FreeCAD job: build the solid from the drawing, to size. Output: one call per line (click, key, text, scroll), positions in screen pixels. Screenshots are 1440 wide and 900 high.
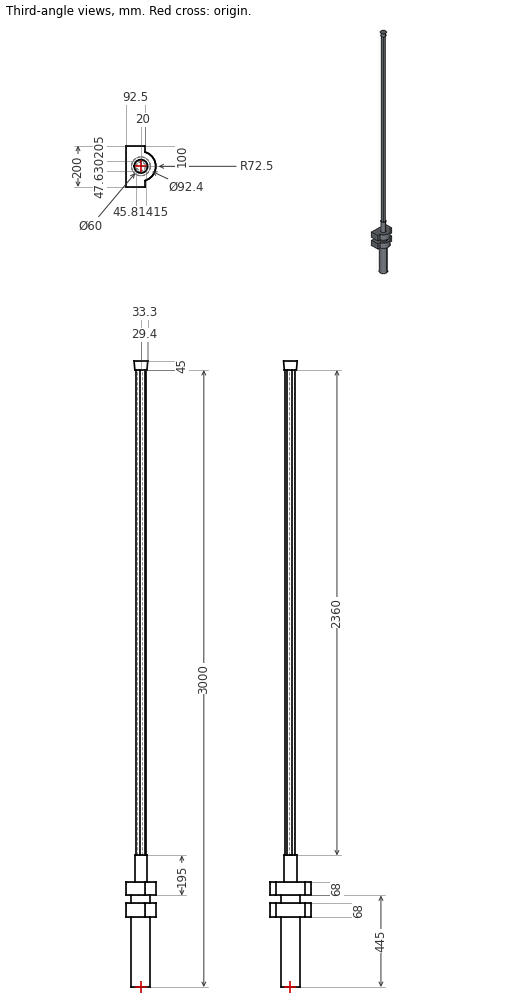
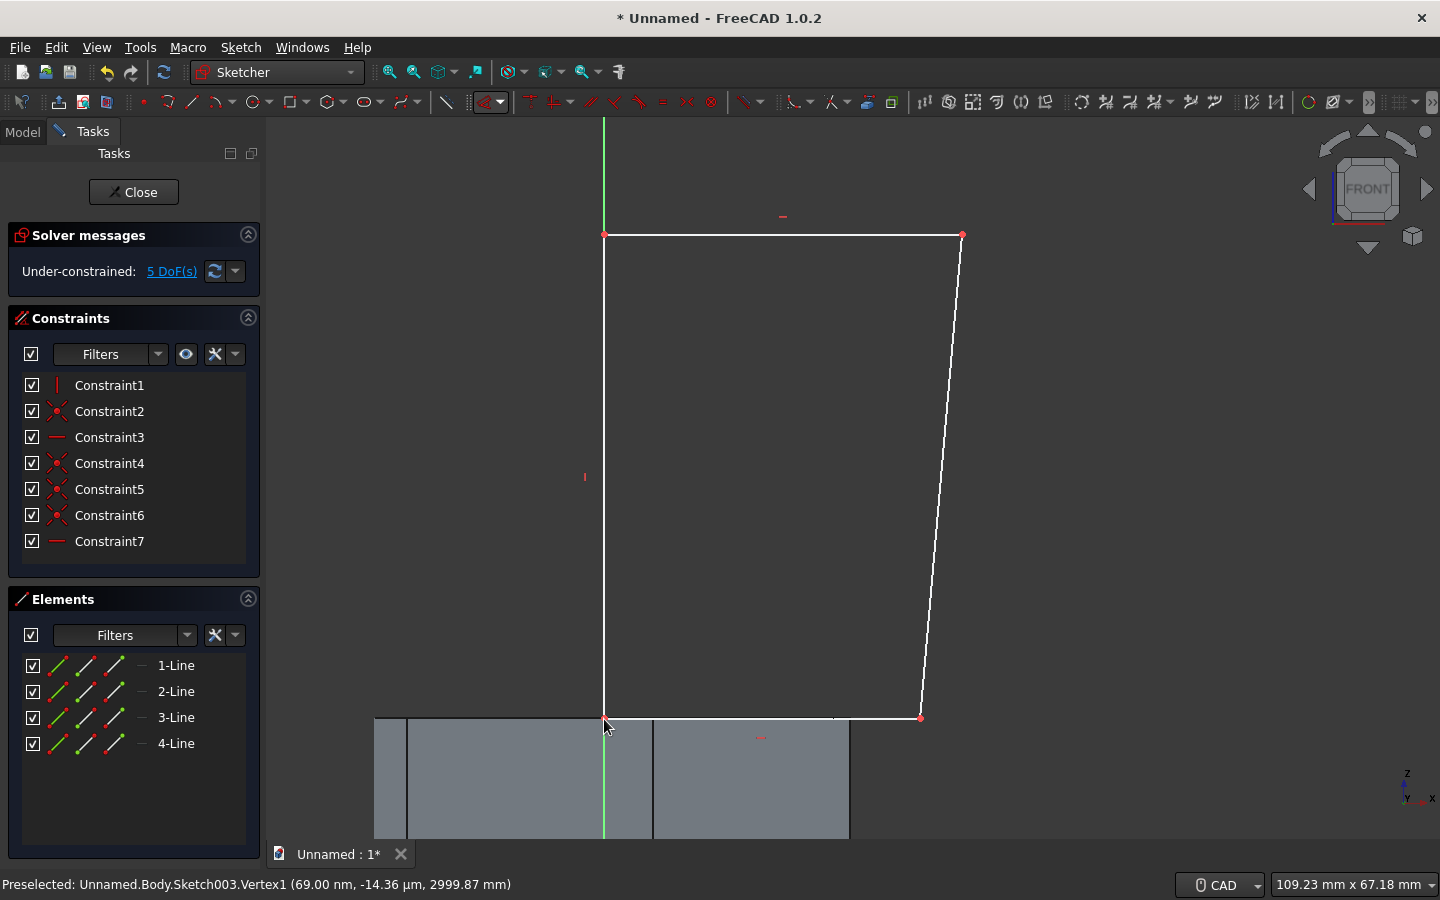
click(604, 719)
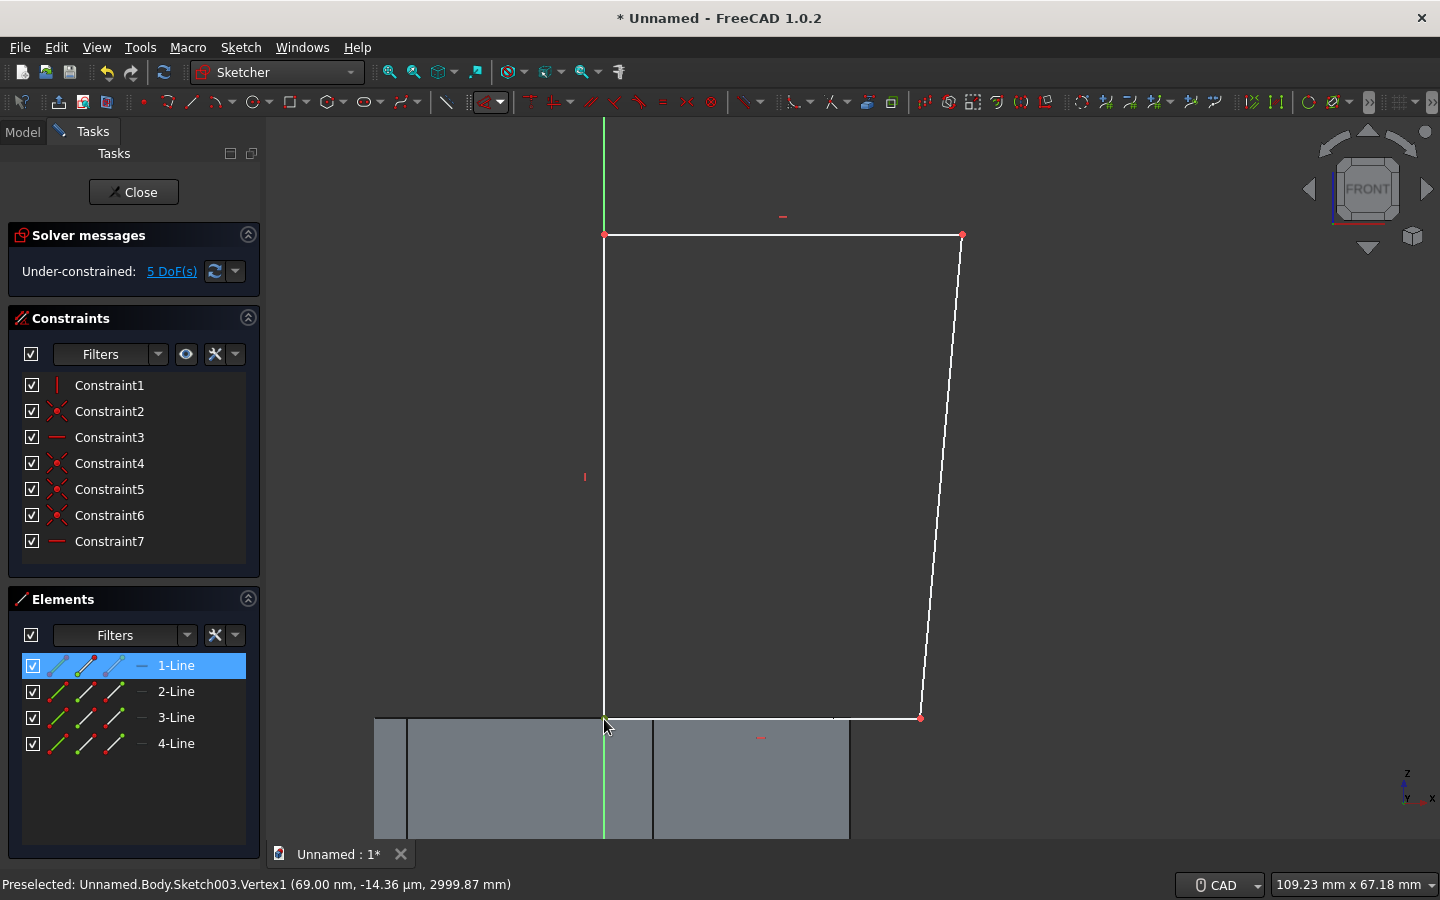
click(604, 763)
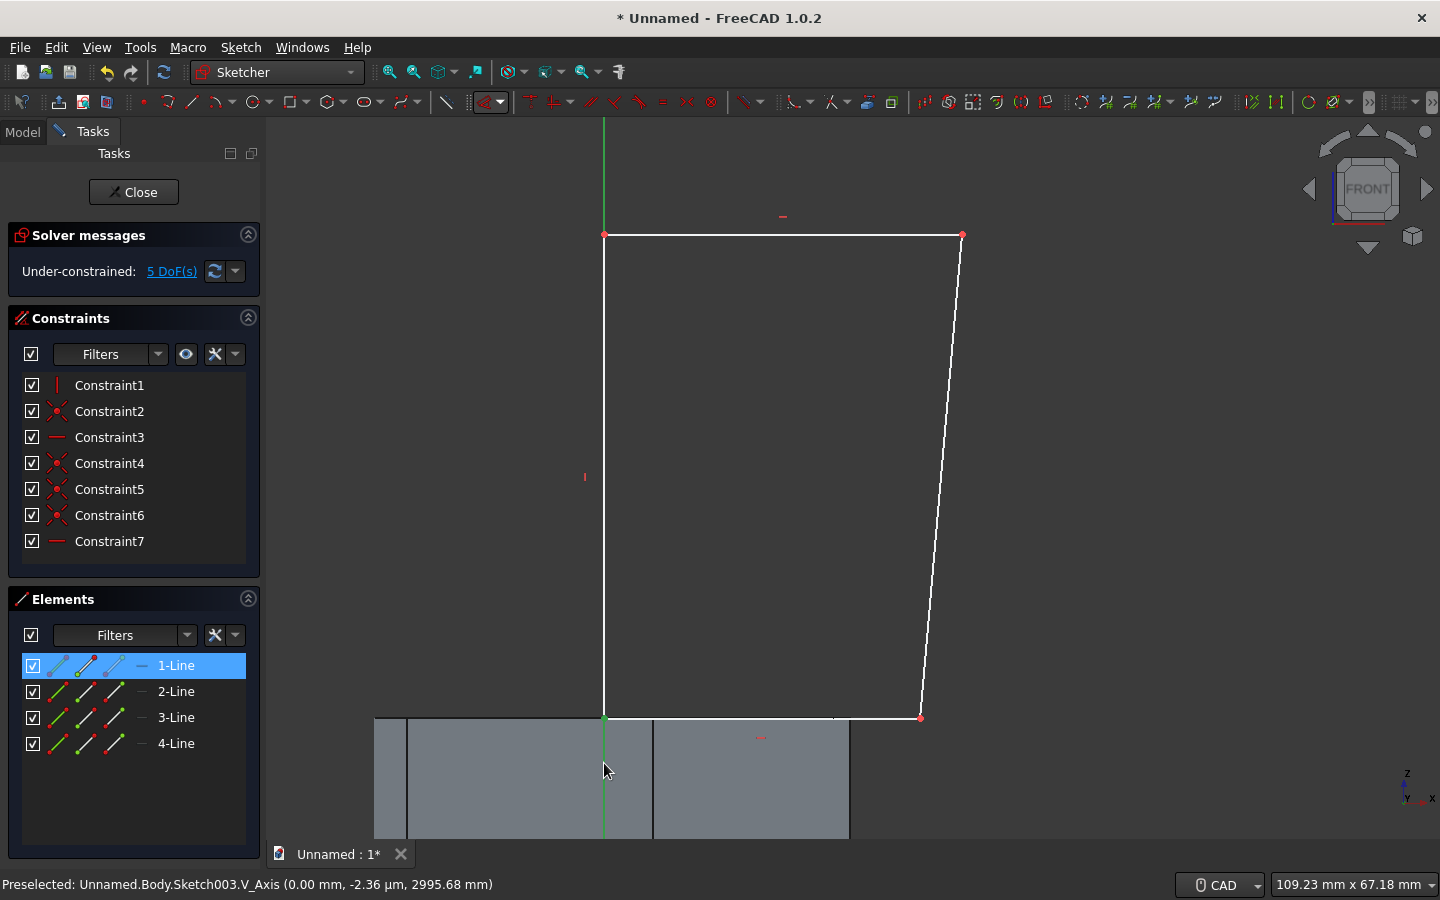
key(c)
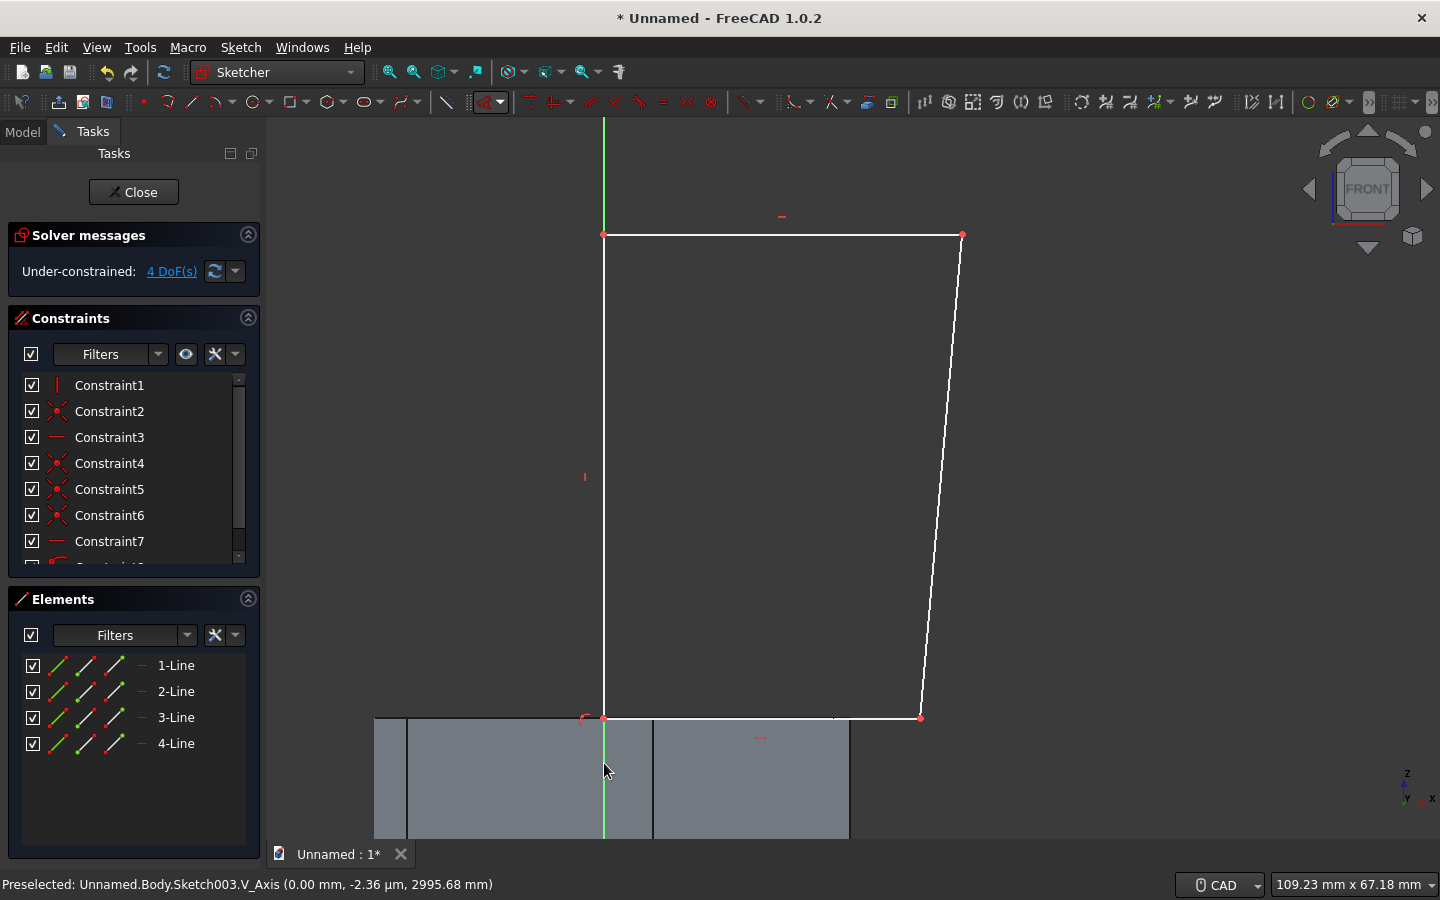
click(604, 574)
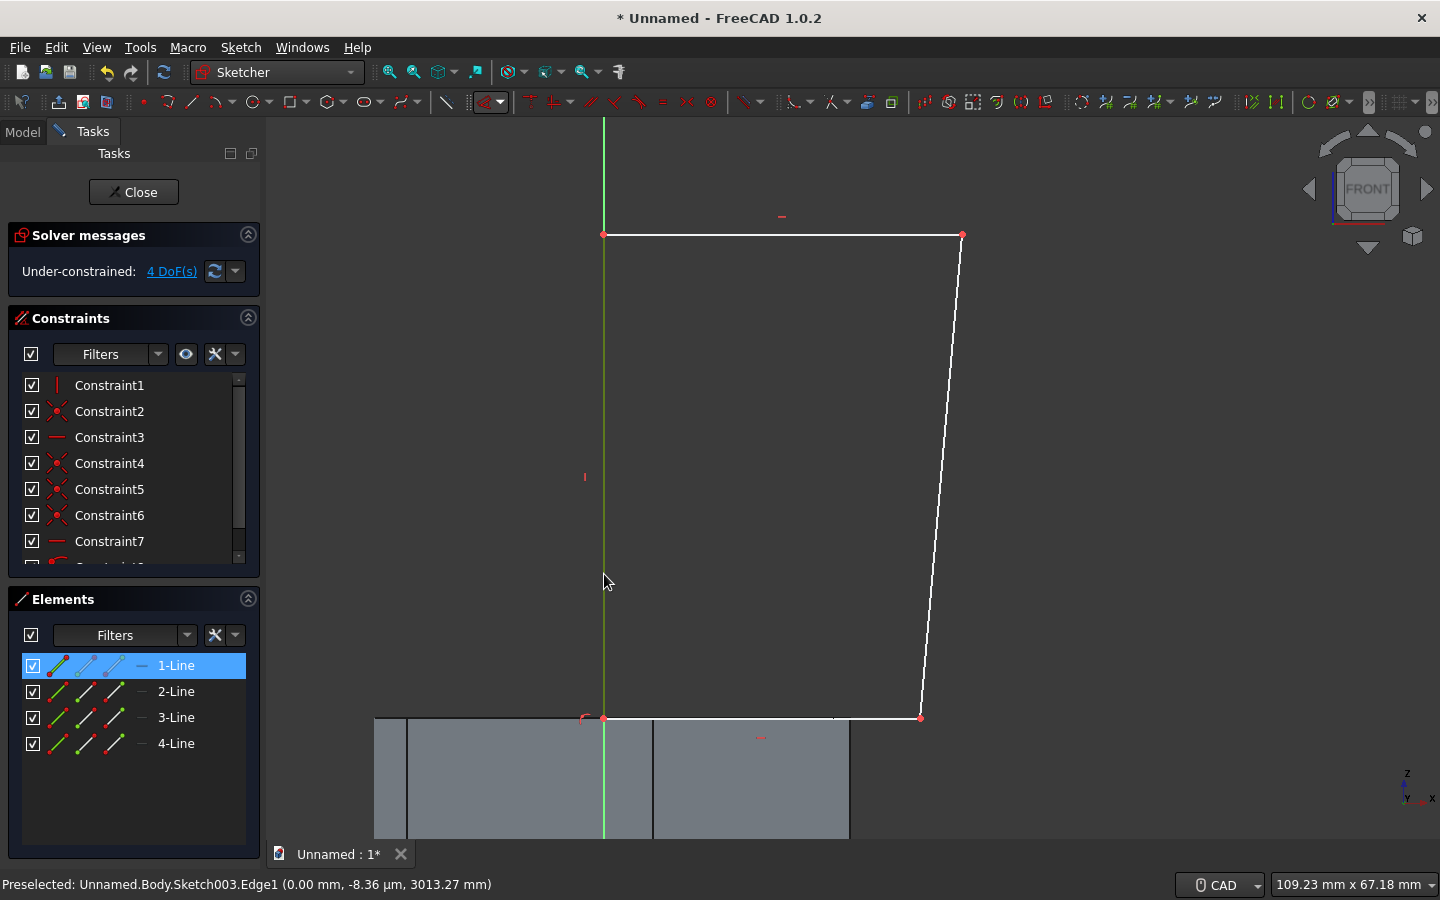
key(i)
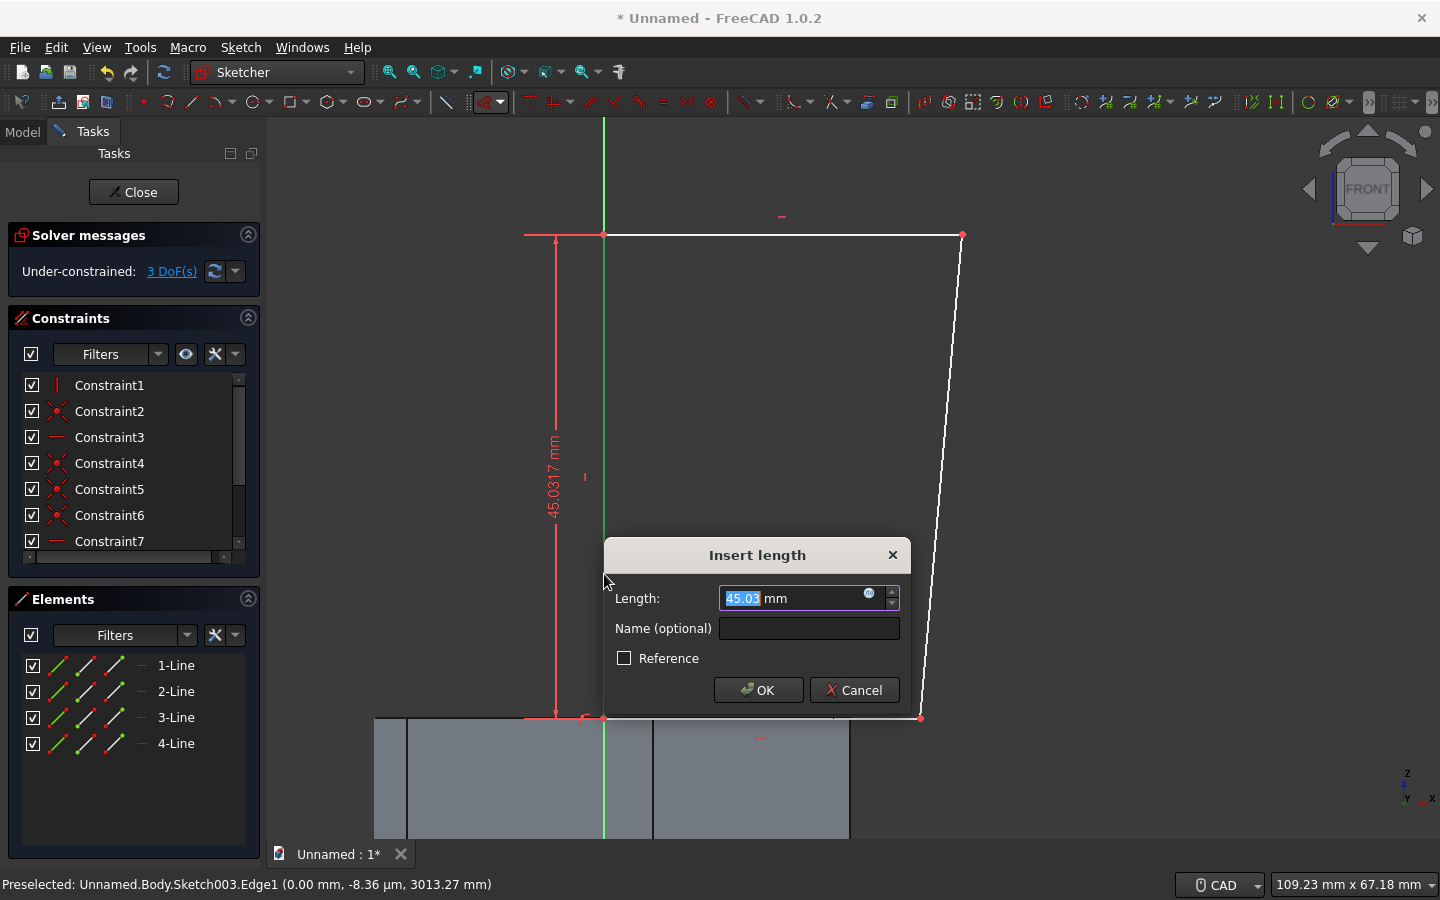
text(45)
key(Return)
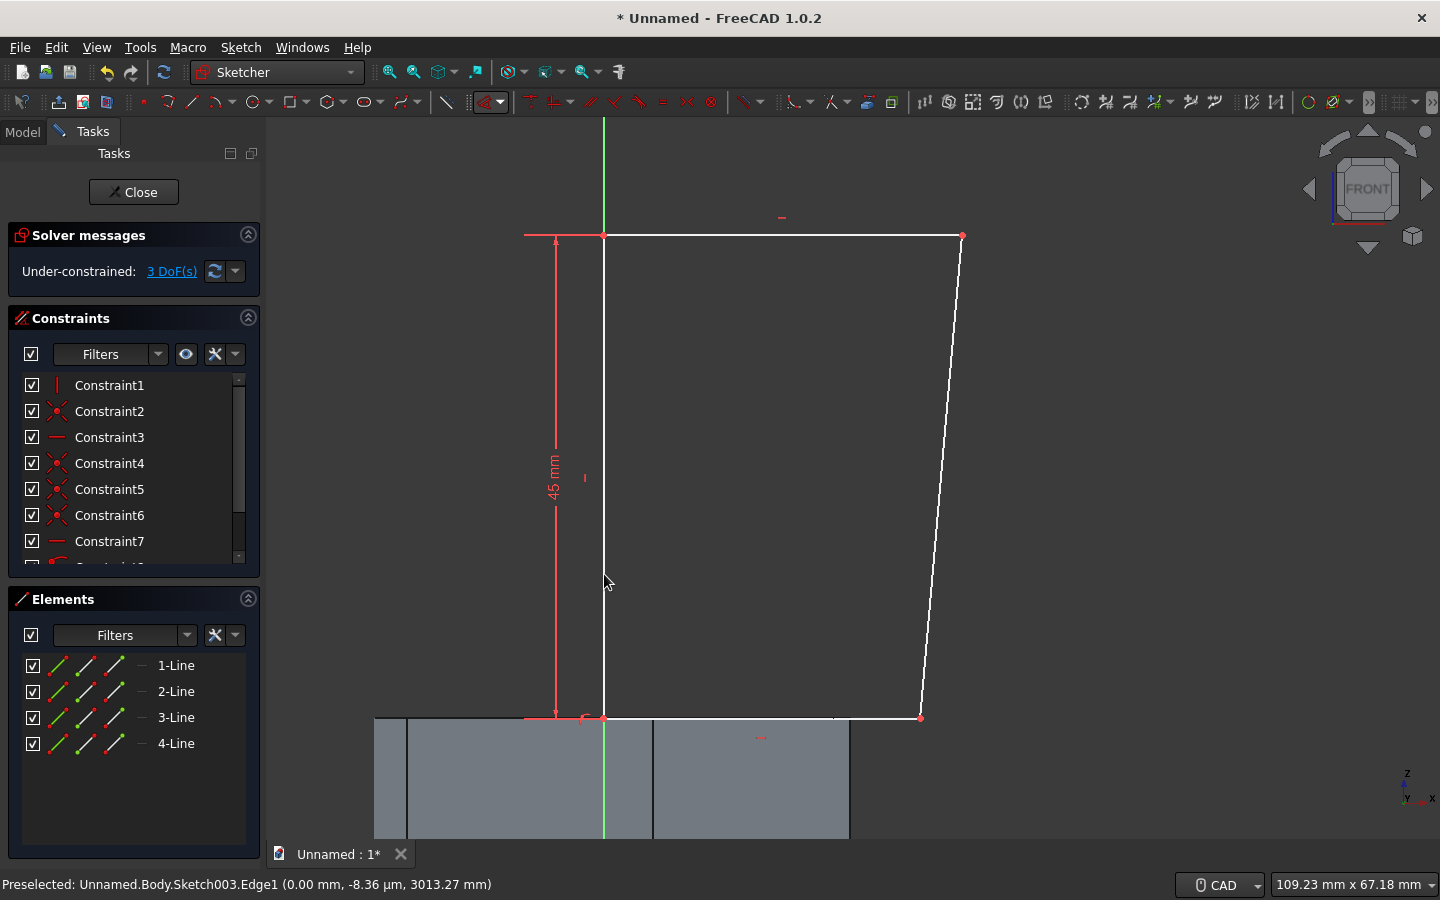
click(711, 235)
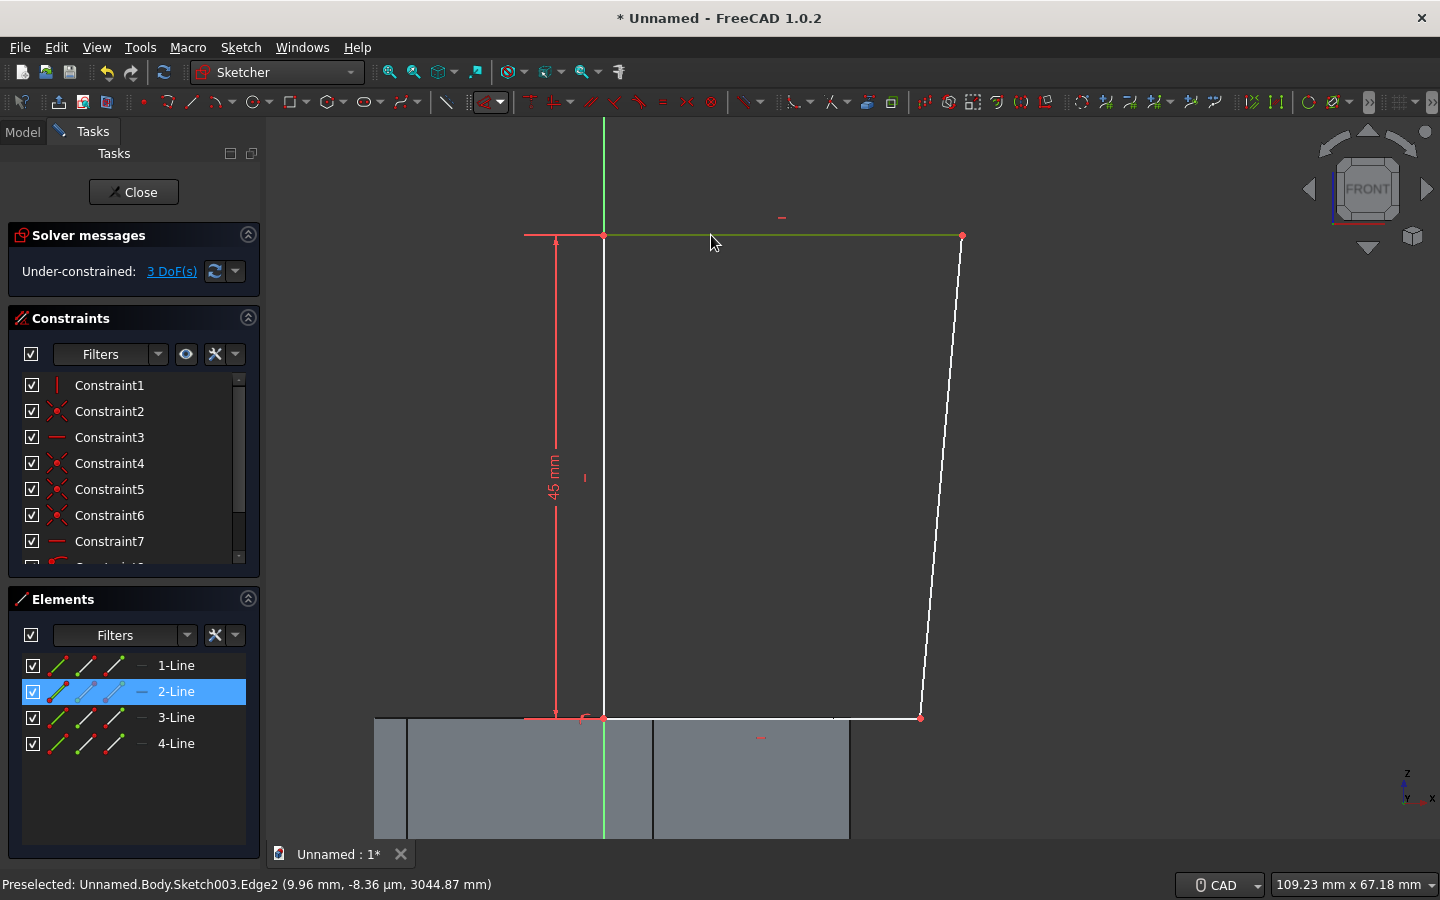
key(l)